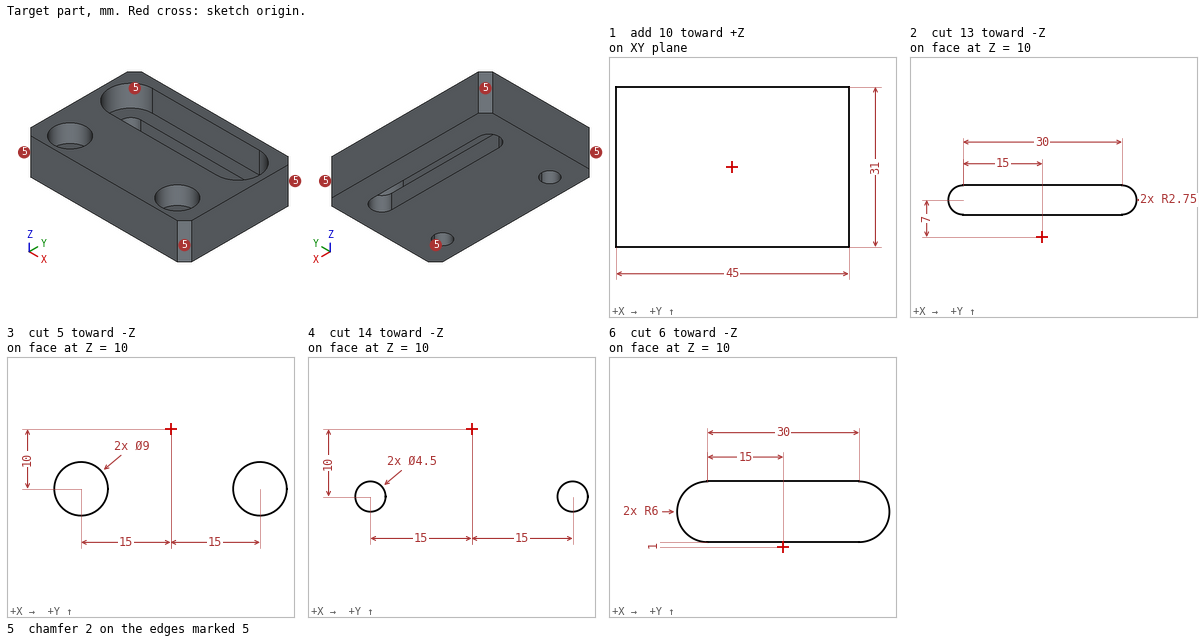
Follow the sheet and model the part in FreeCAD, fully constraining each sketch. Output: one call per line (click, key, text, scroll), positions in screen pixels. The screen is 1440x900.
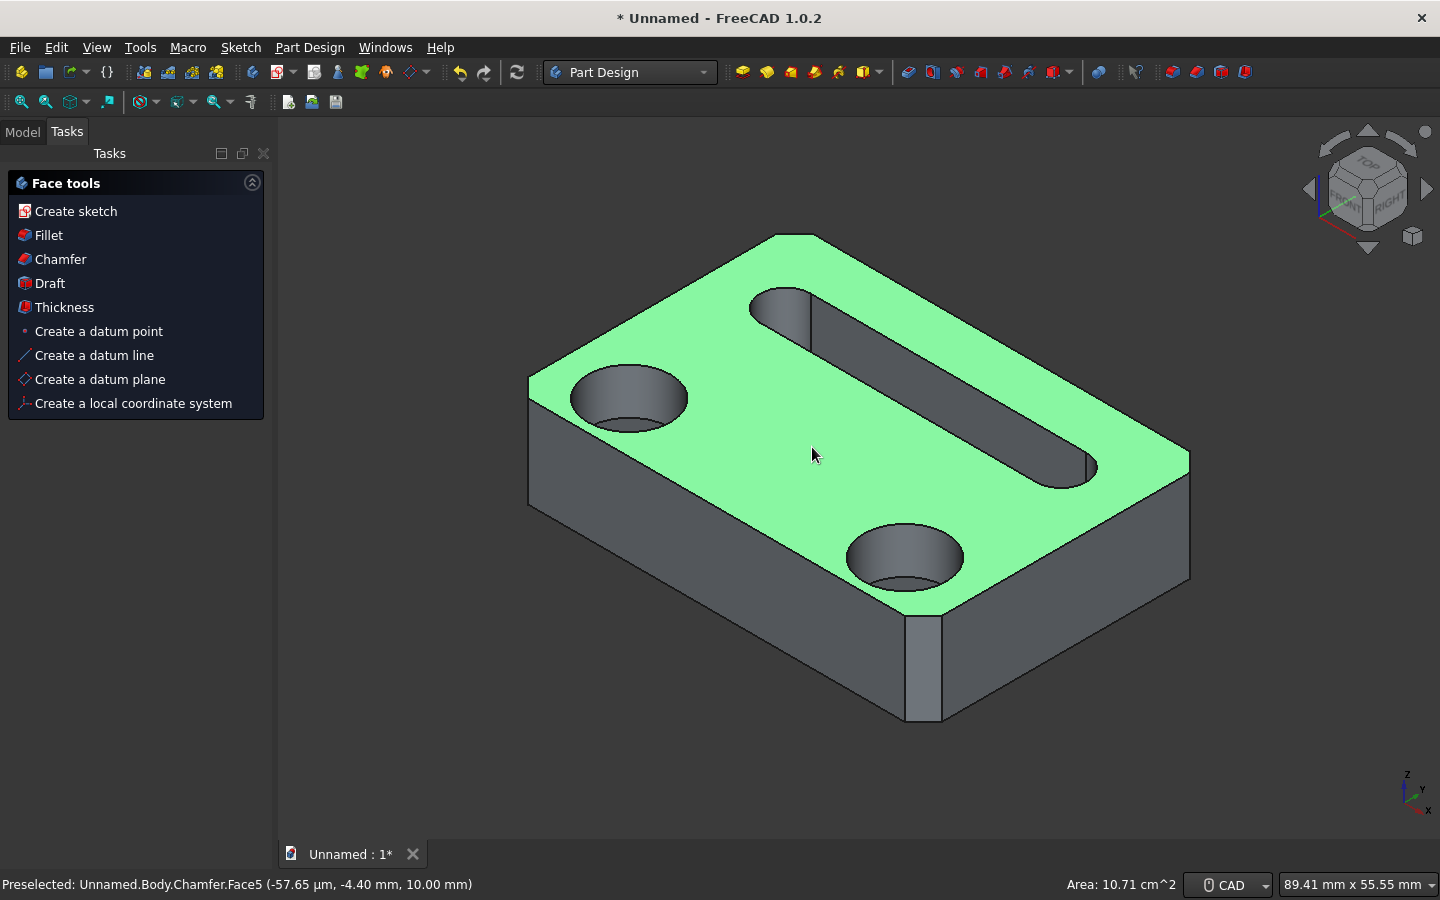
click(278, 72)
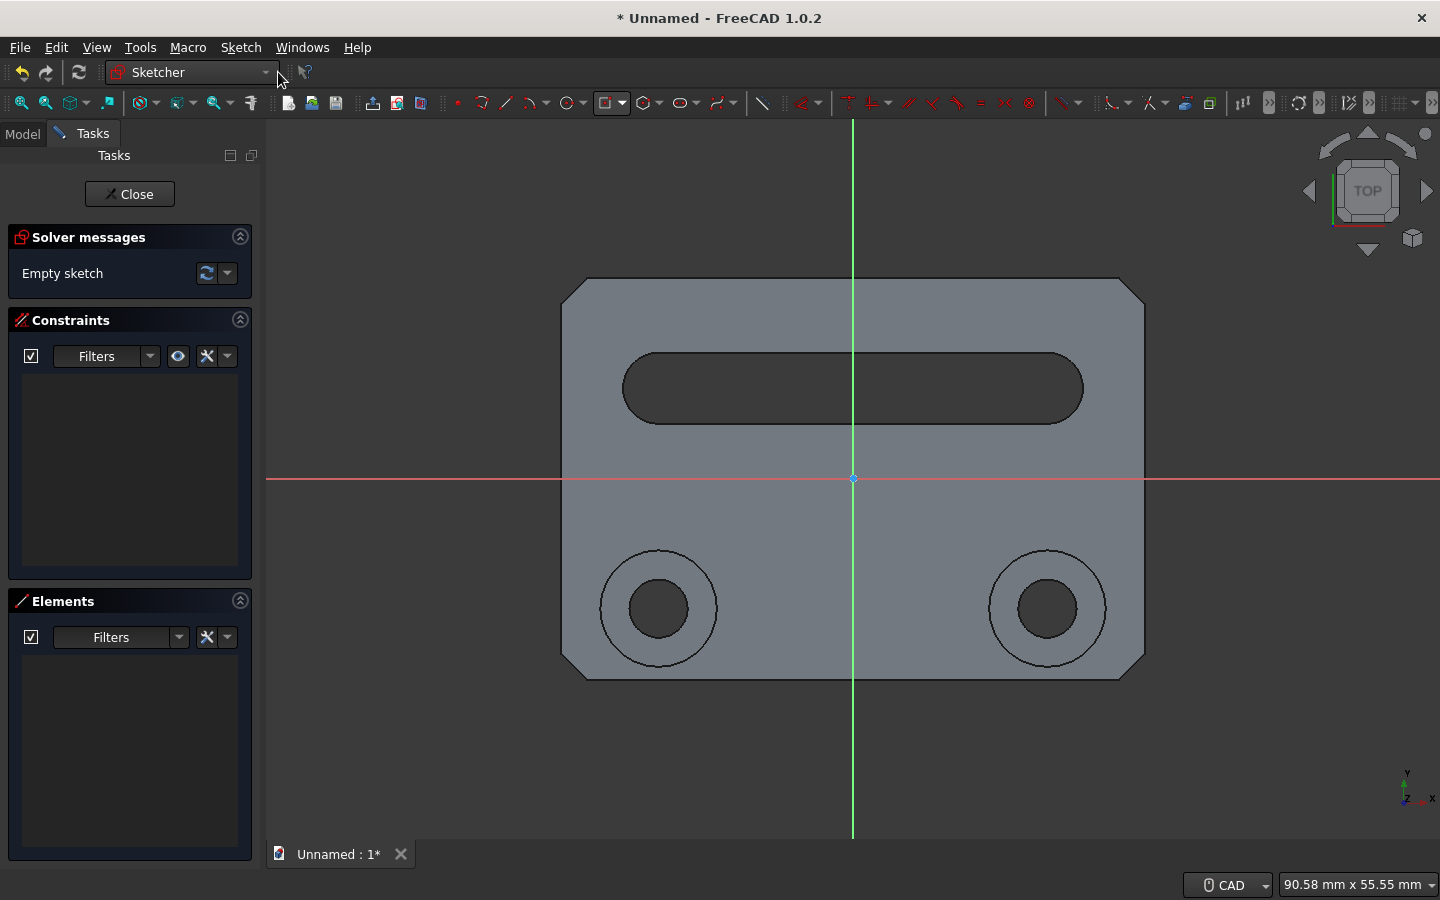
click(680, 104)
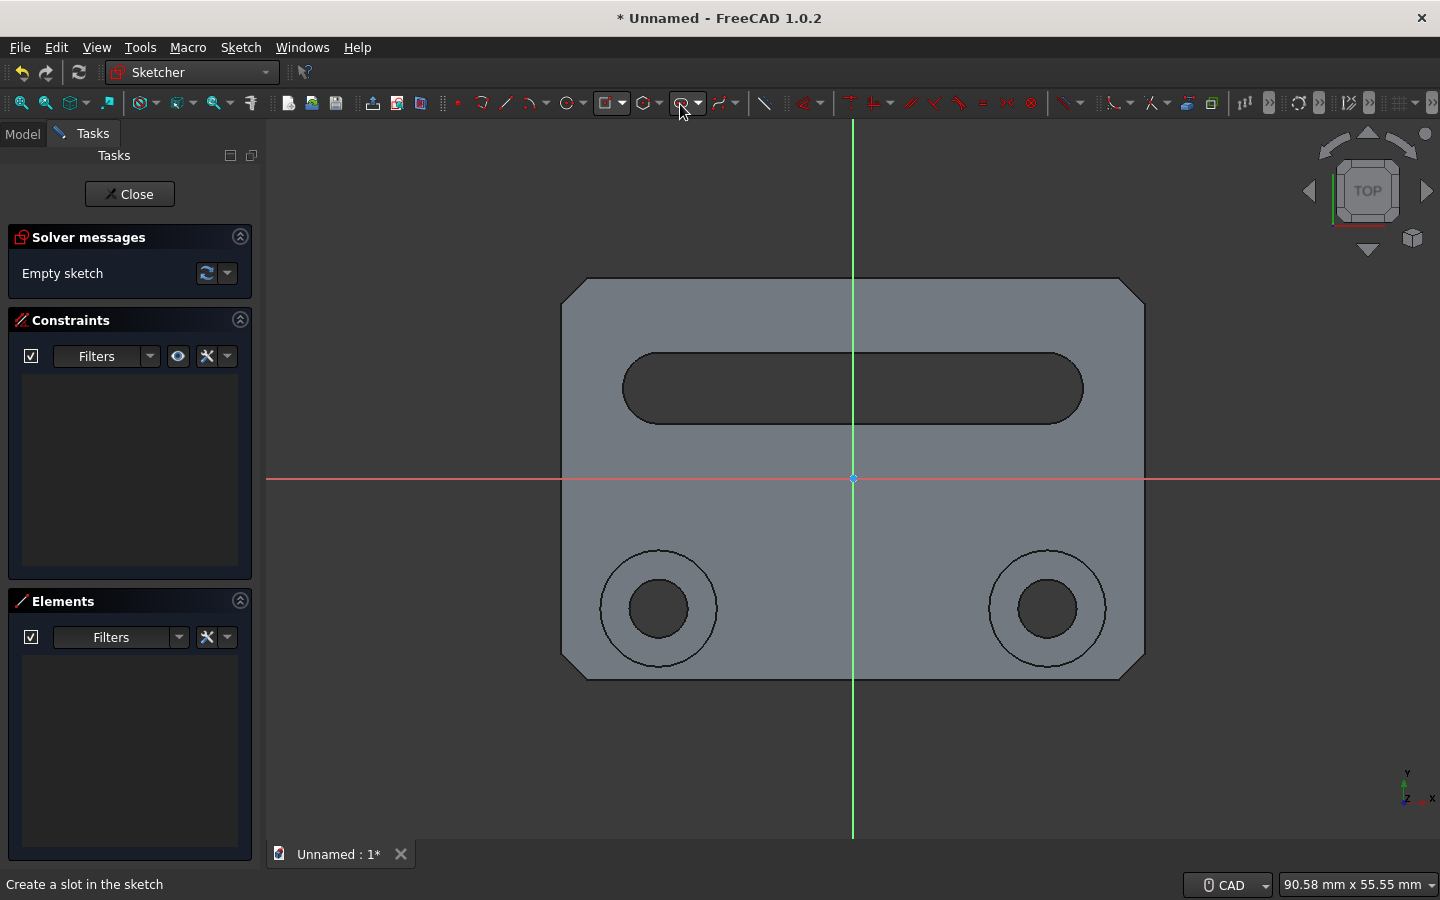
click(659, 388)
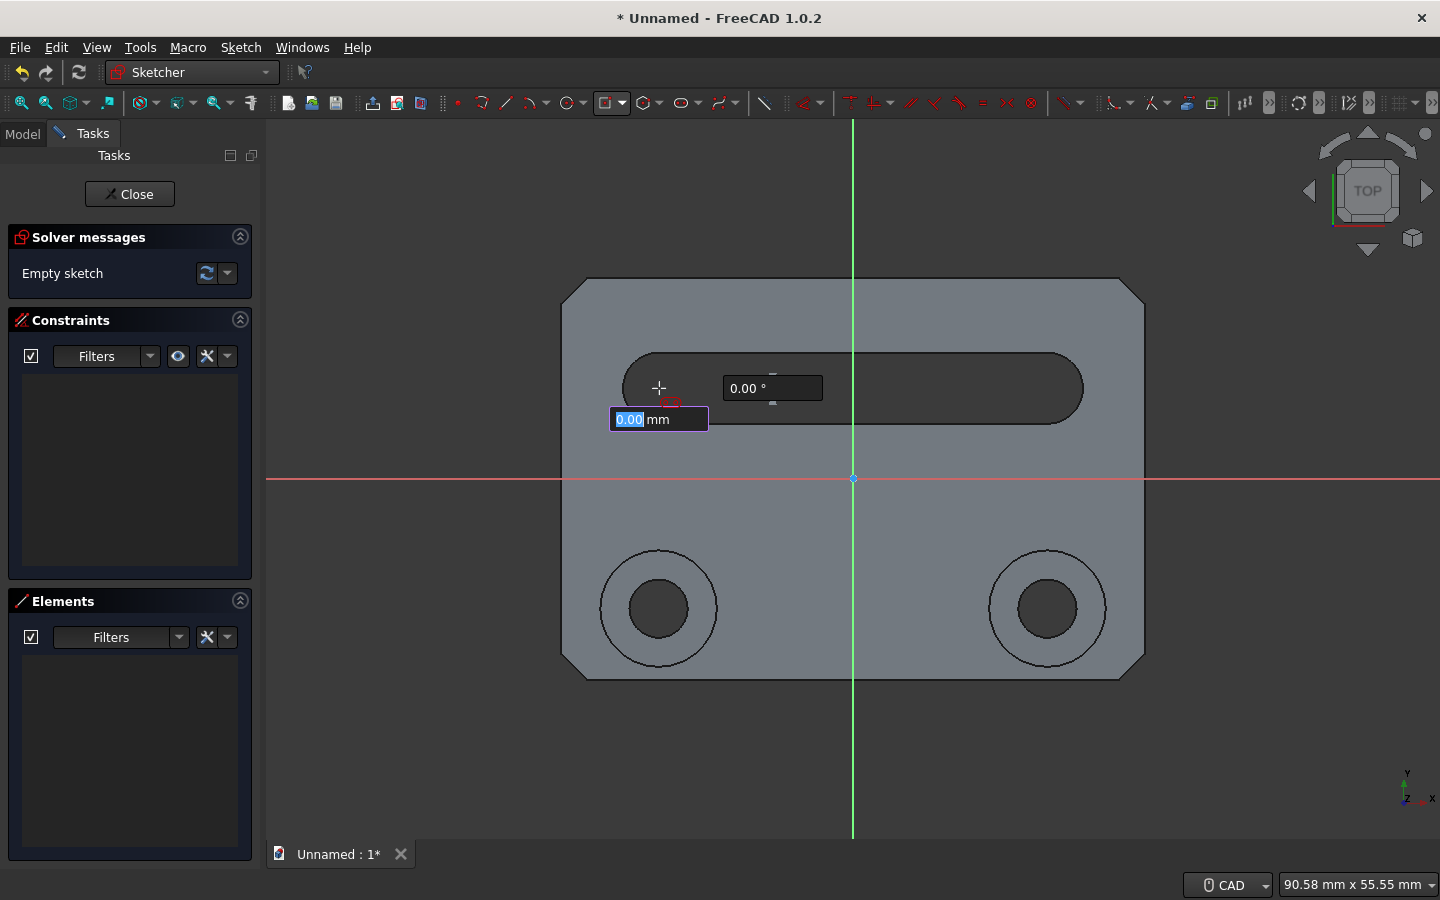
click(1047, 388)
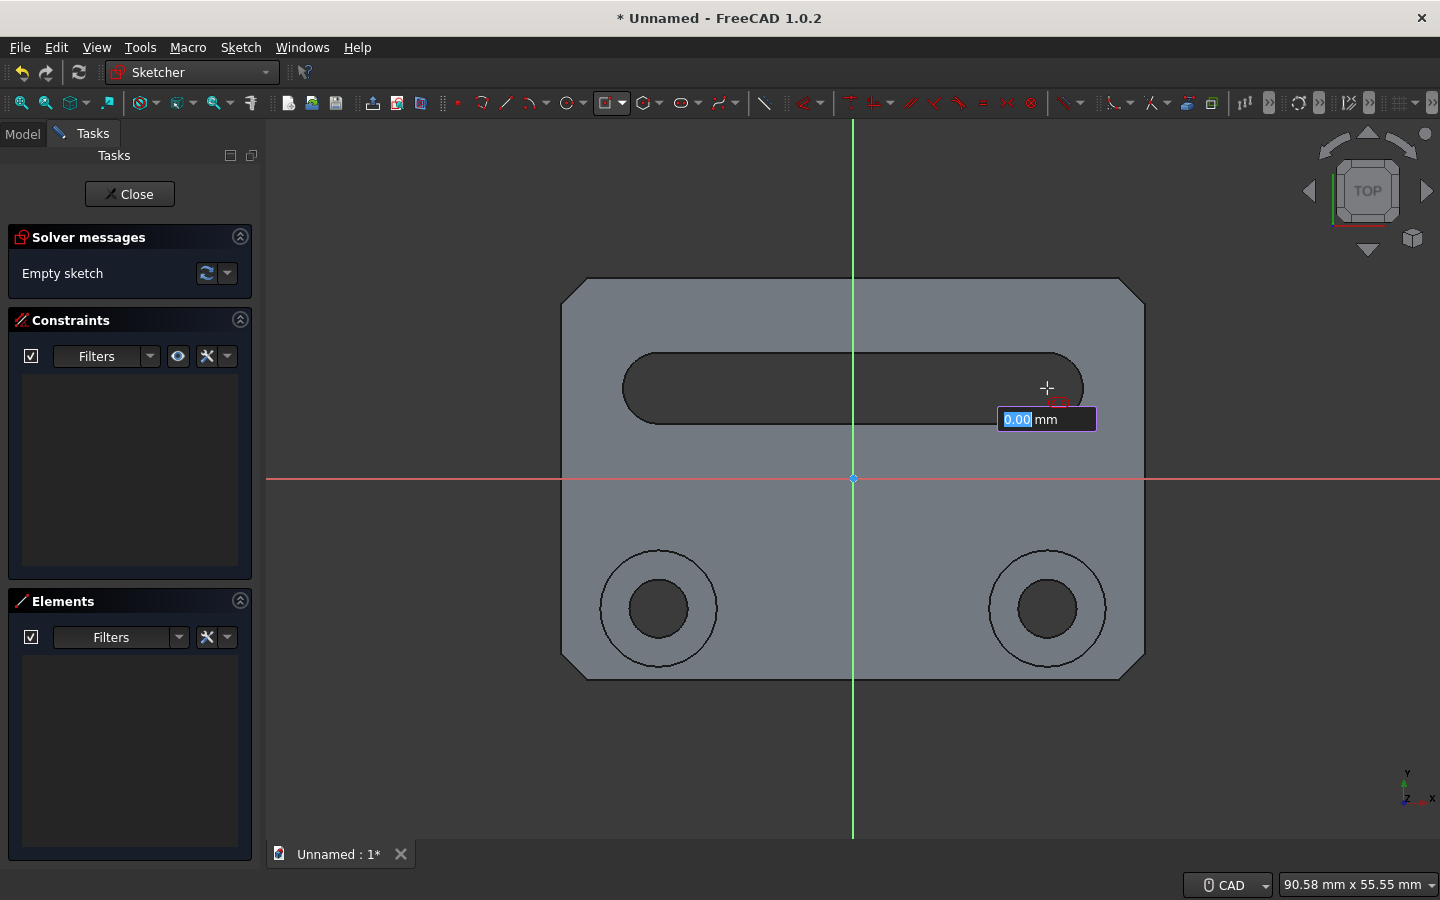
click(911, 311)
key(Escape)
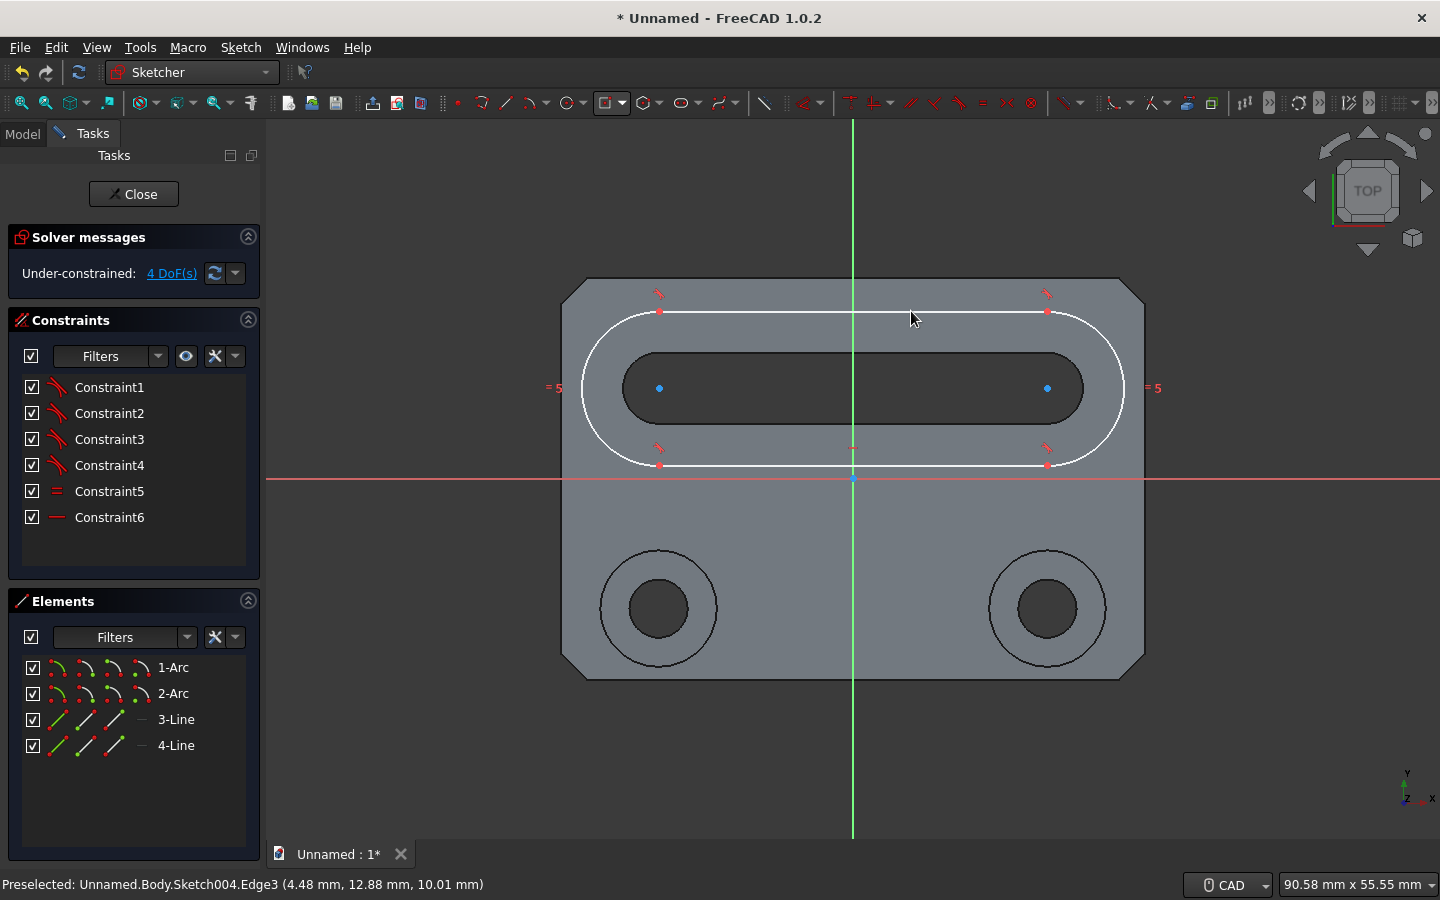
click(804, 104)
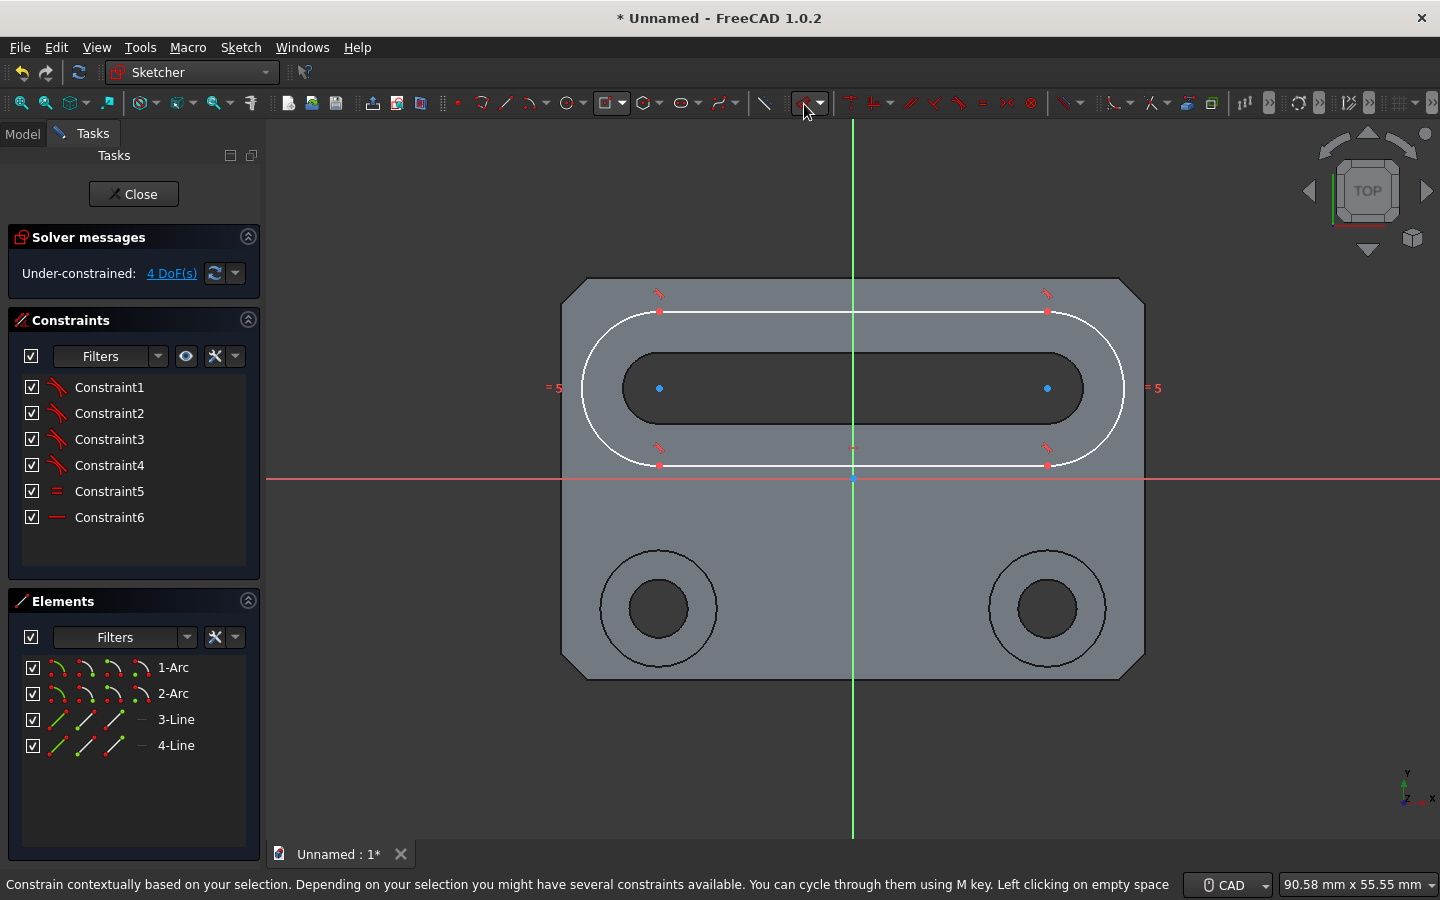
click(597, 344)
click(571, 325)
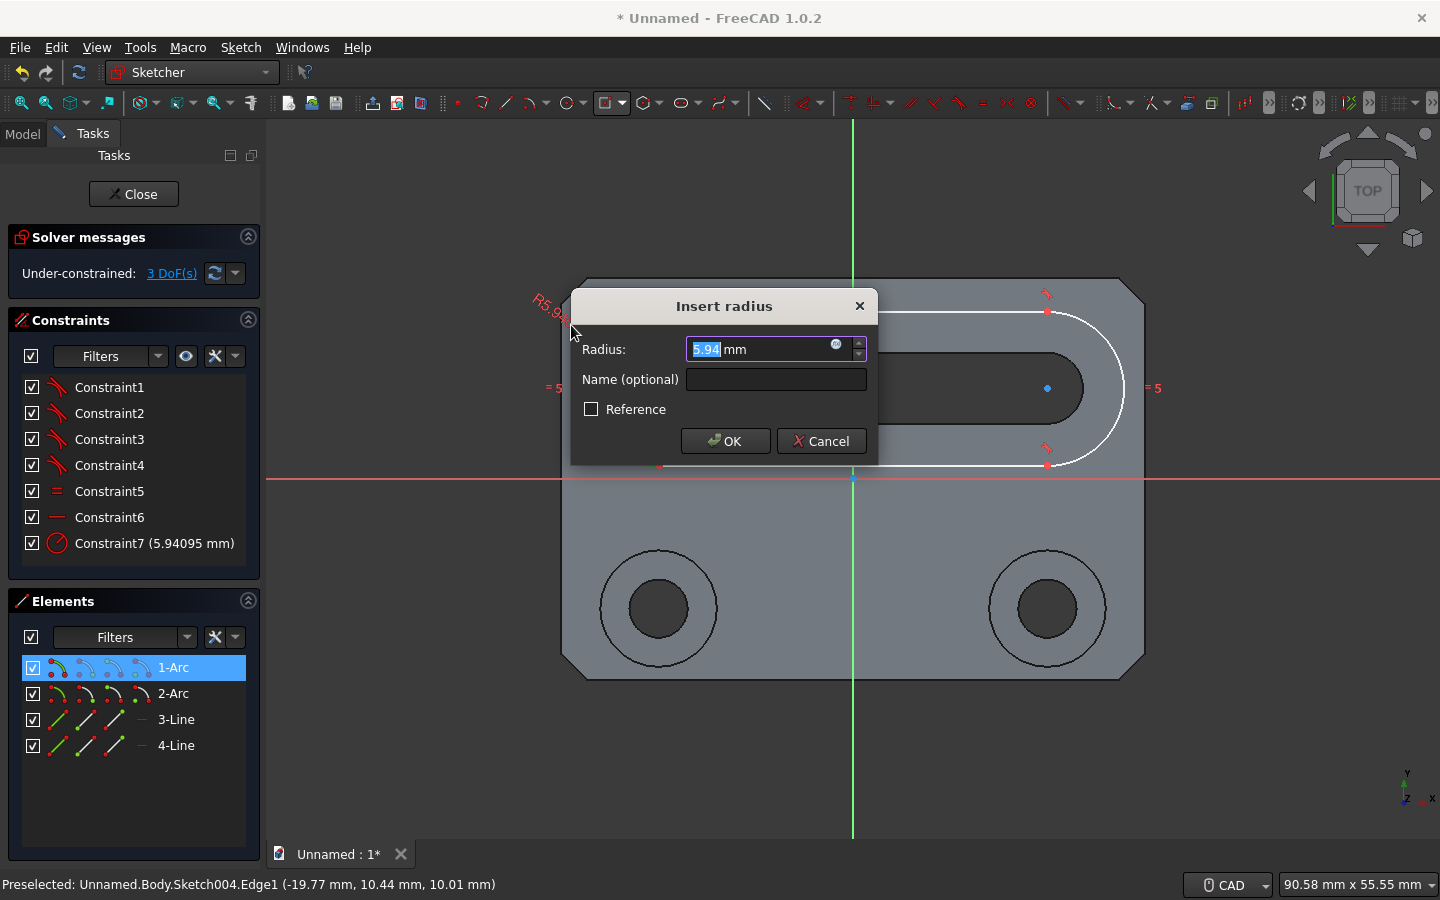
text(6)
key(Return)